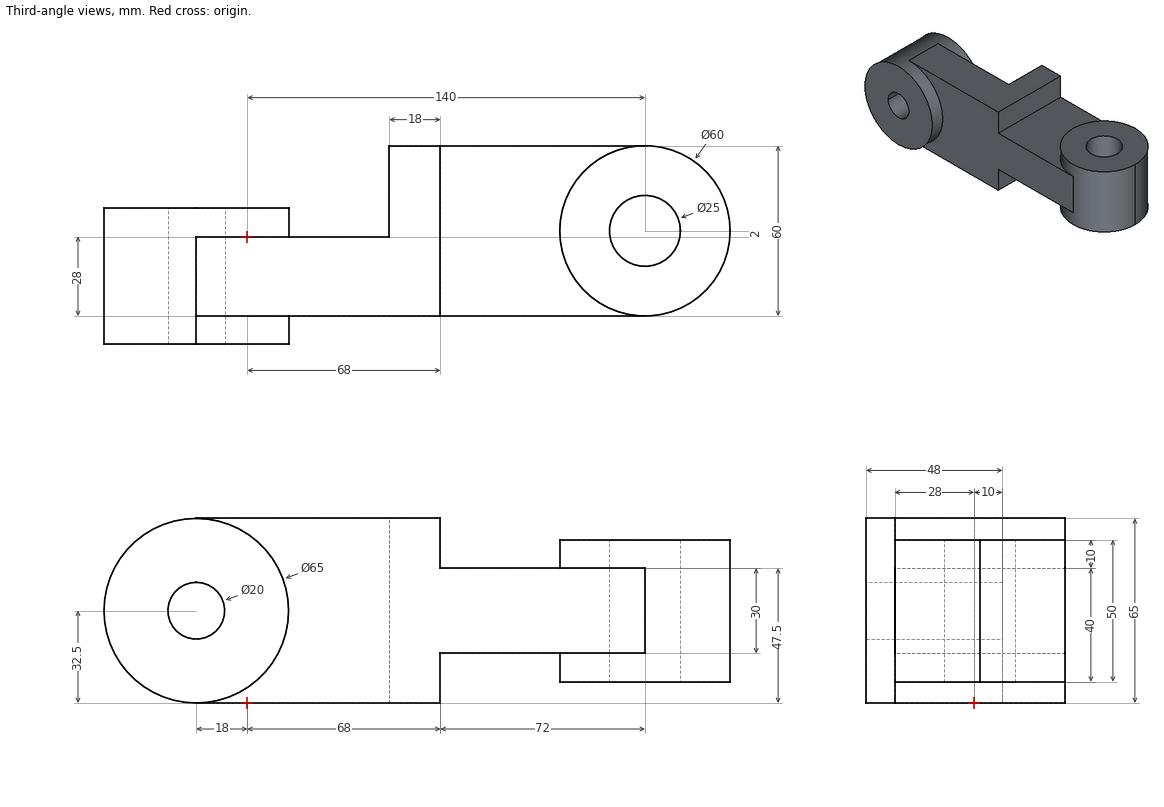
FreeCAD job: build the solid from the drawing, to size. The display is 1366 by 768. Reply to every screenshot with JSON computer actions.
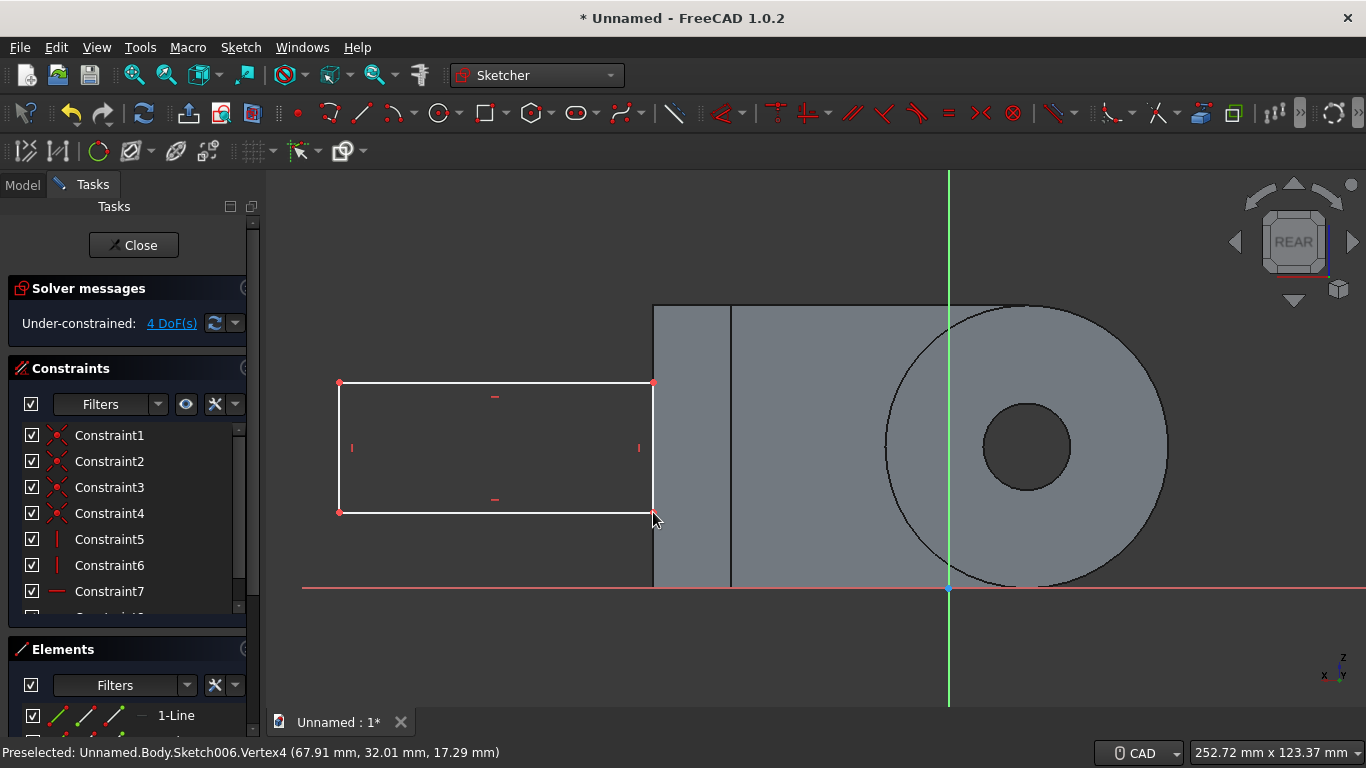
{"action": "key", "text": "d"}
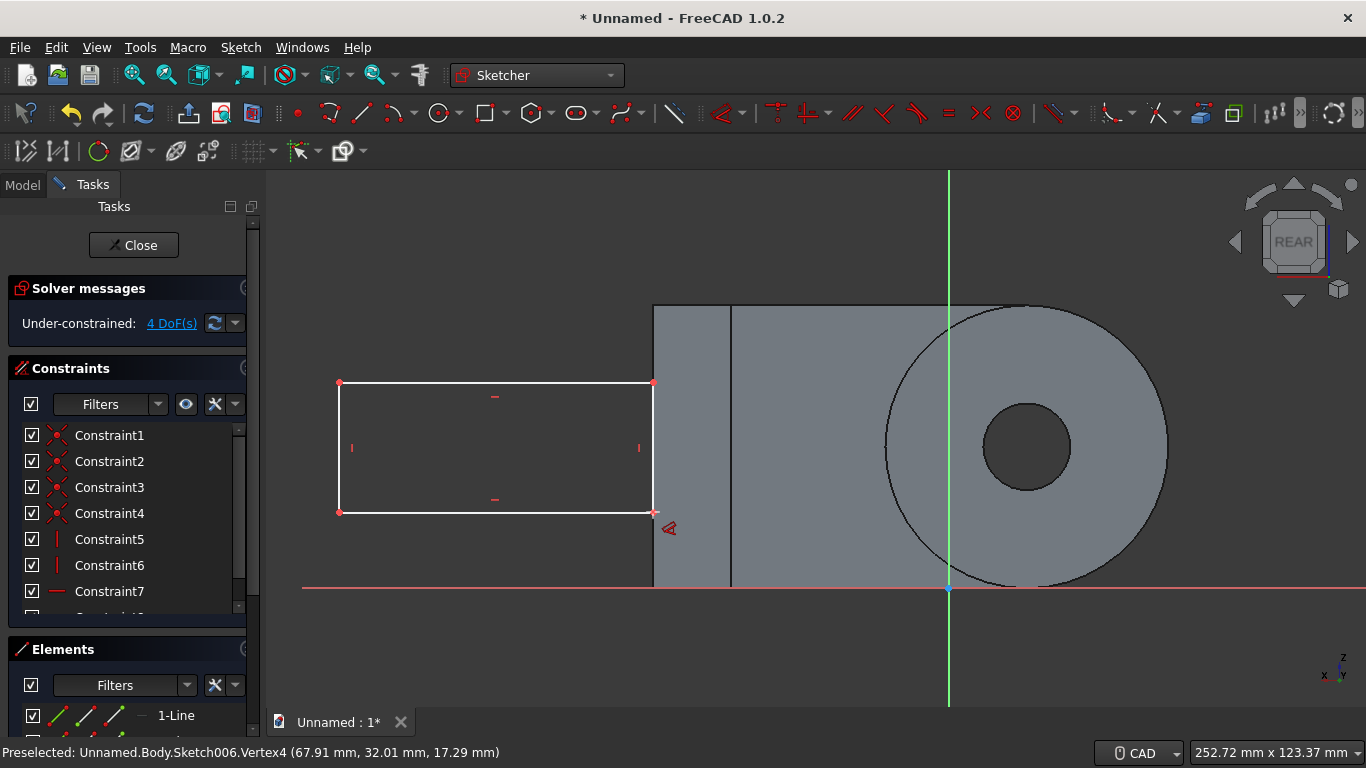
{"action": "left_click", "coordinate": [339, 422]}
{"action": "left_click", "coordinate": [305, 448]}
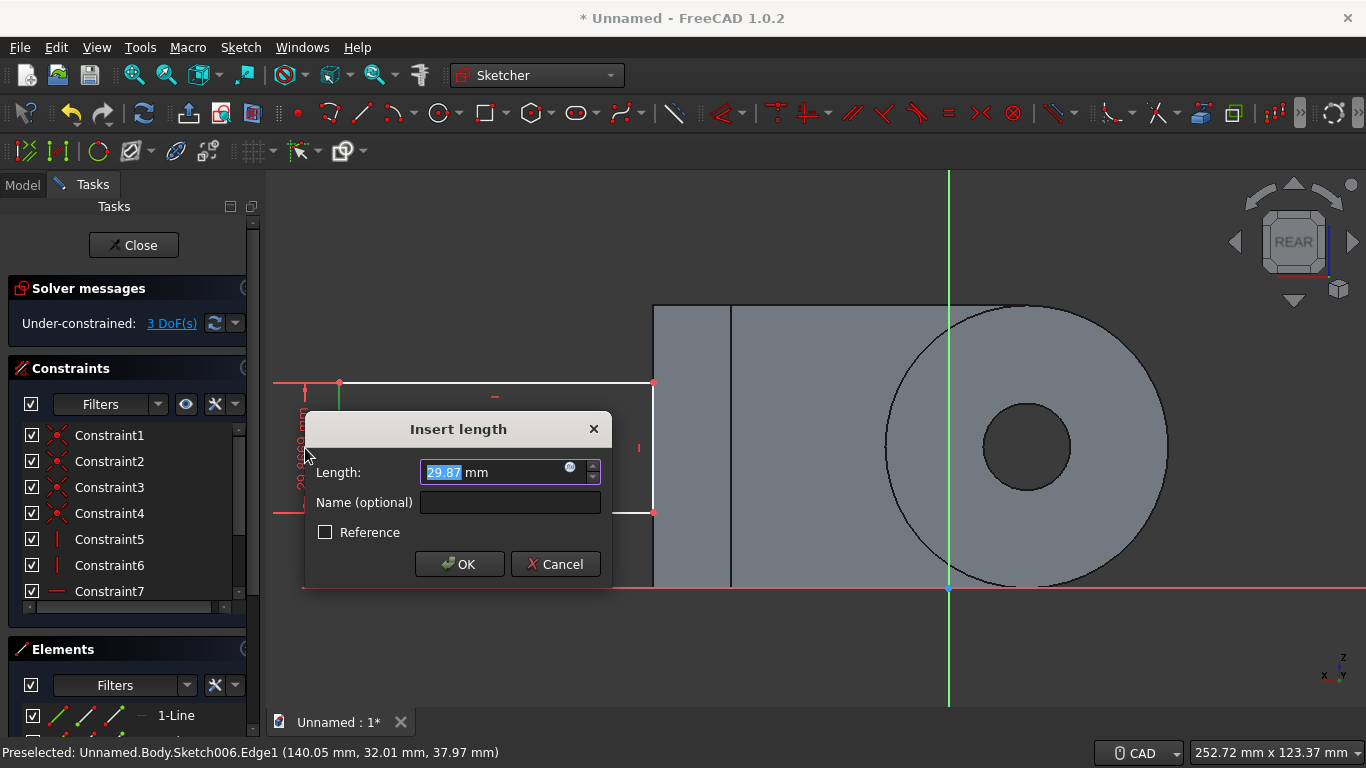
{"action": "type", "text": "30"}
{"action": "key", "text": "Return"}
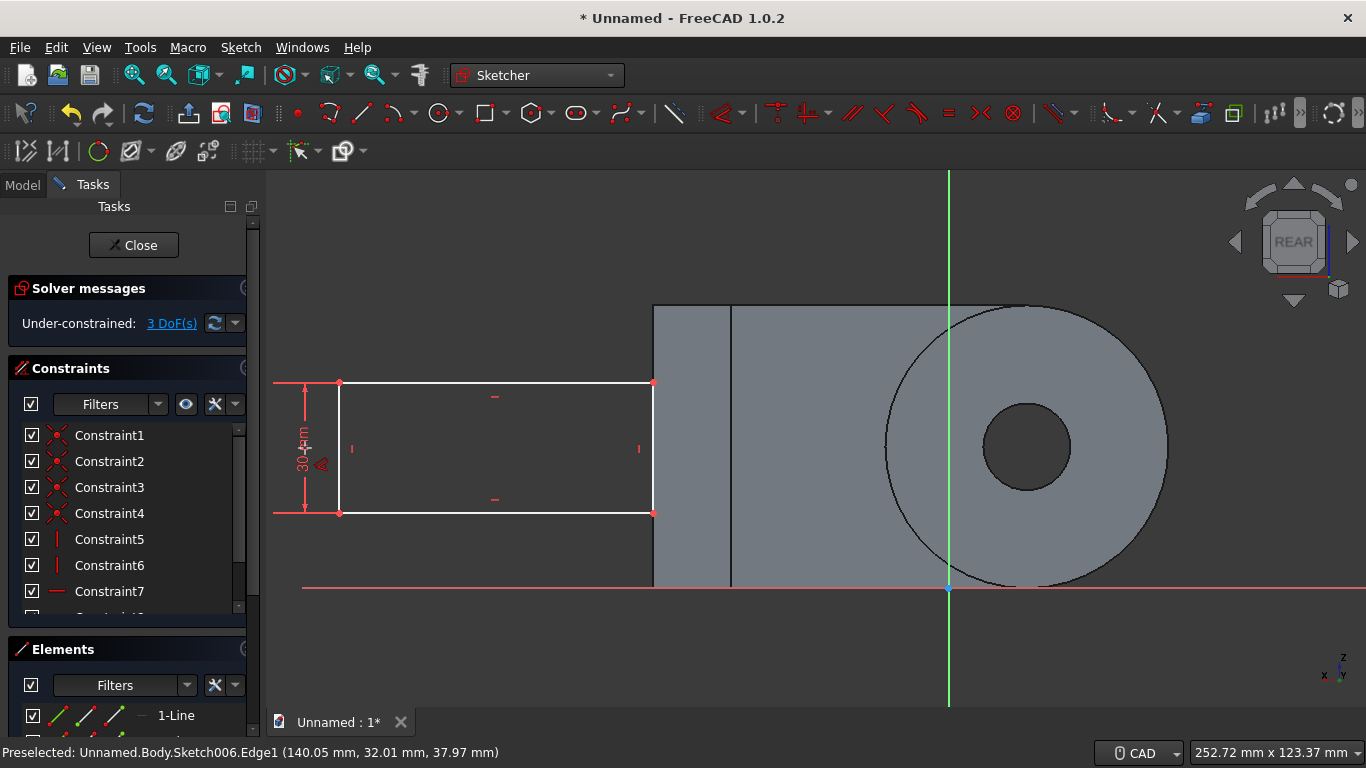
{"action": "left_click", "coordinate": [433, 513]}
{"action": "left_click", "coordinate": [496, 547]}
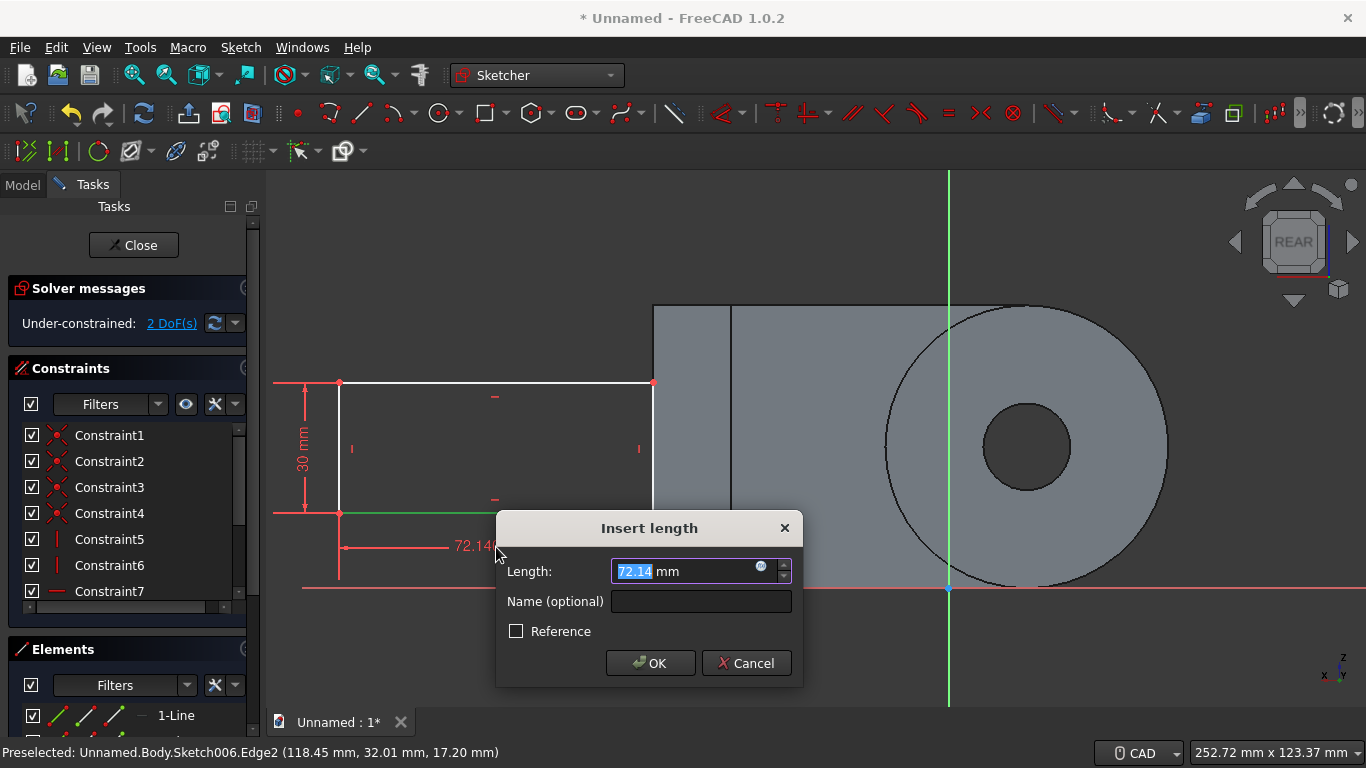
{"action": "type", "text": "72"}
{"action": "key", "text": "Return"}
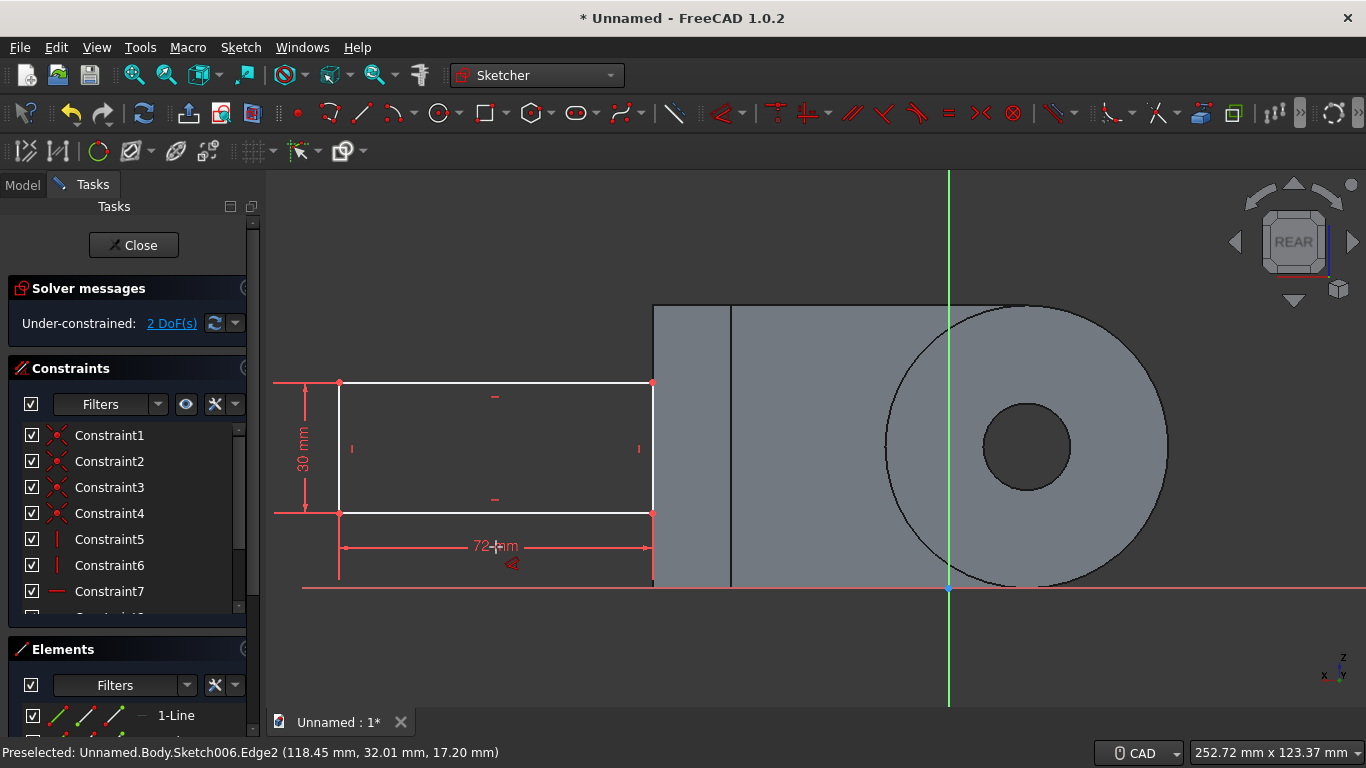
{"action": "left_click", "coordinate": [653, 513]}
{"action": "left_click", "coordinate": [801, 622]}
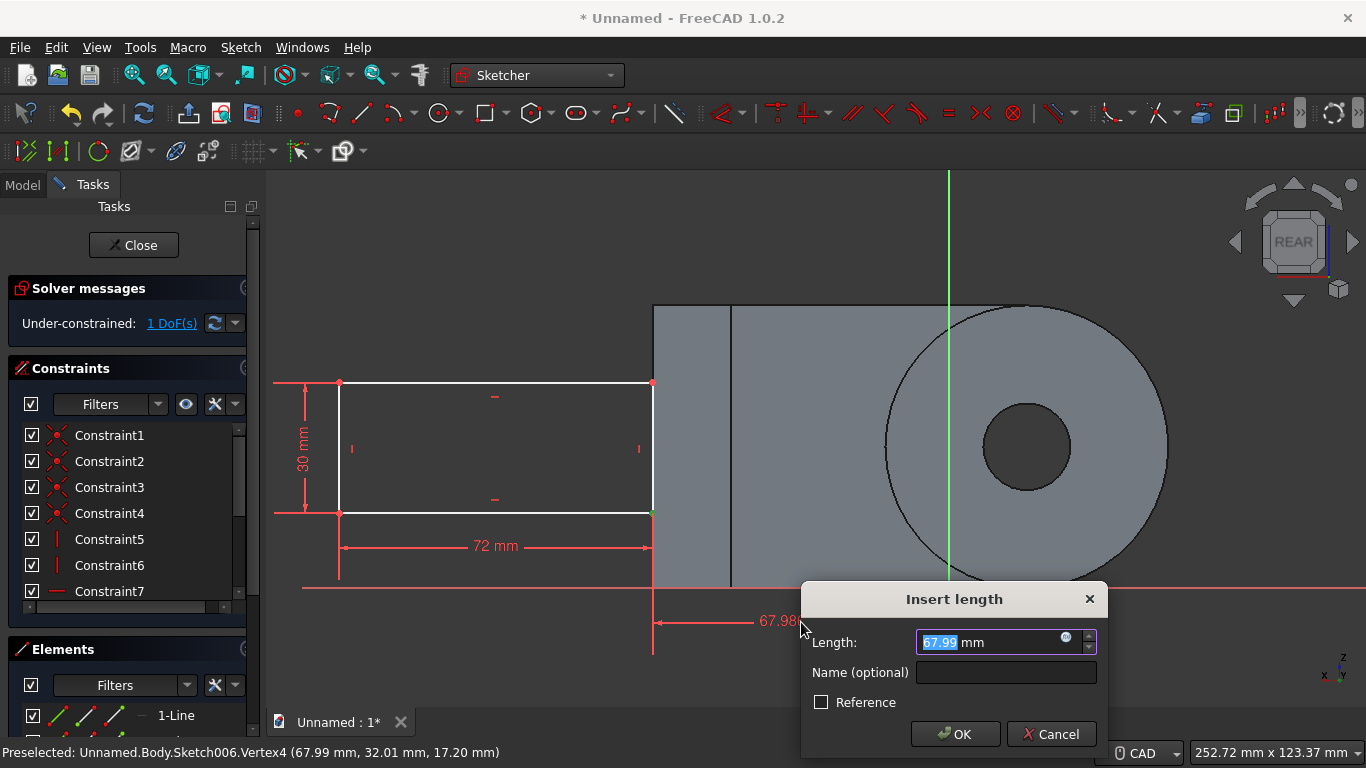
{"action": "type", "text": "68"}
{"action": "key", "text": "Return"}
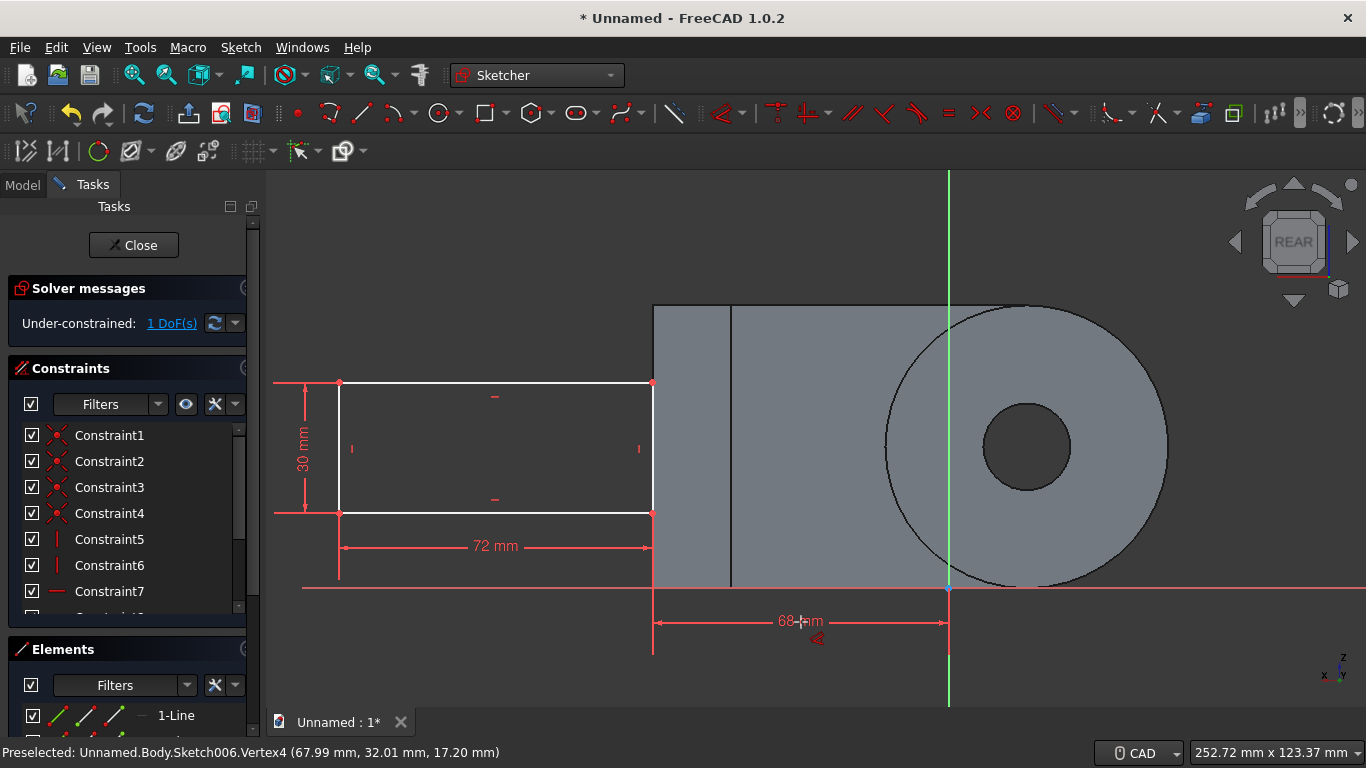
{"action": "left_click", "coordinate": [339, 383]}
{"action": "left_click", "coordinate": [983, 486]}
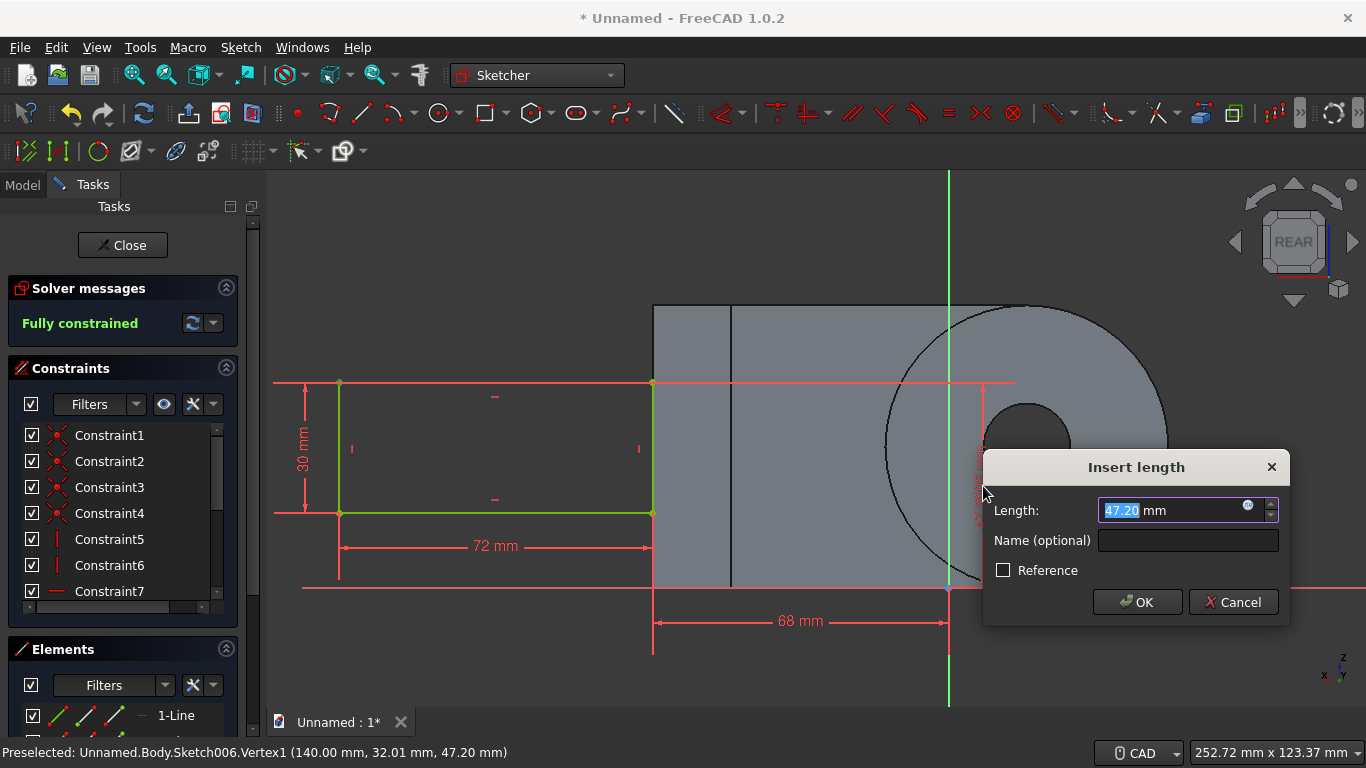
{"action": "type", "text": "47.5"}
{"action": "key", "text": "Return"}
{"action": "key", "text": "Escape"}